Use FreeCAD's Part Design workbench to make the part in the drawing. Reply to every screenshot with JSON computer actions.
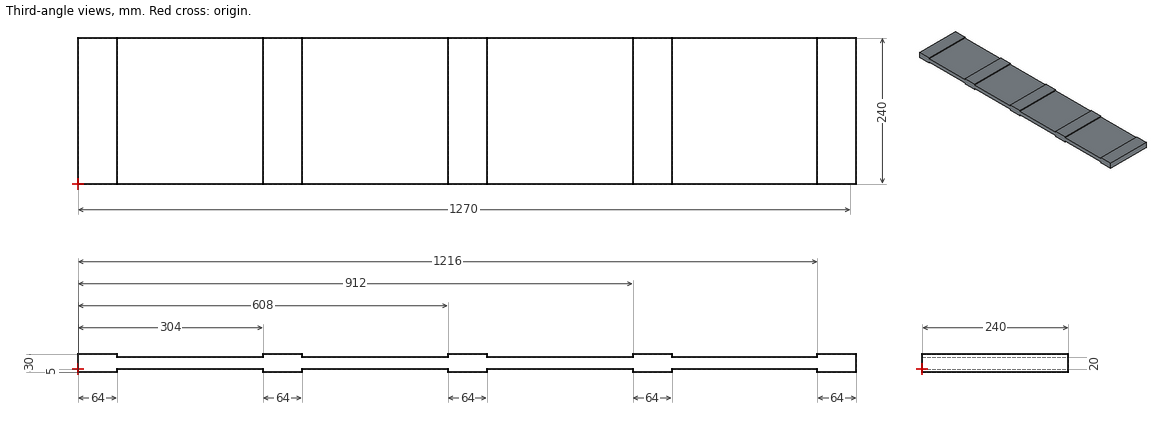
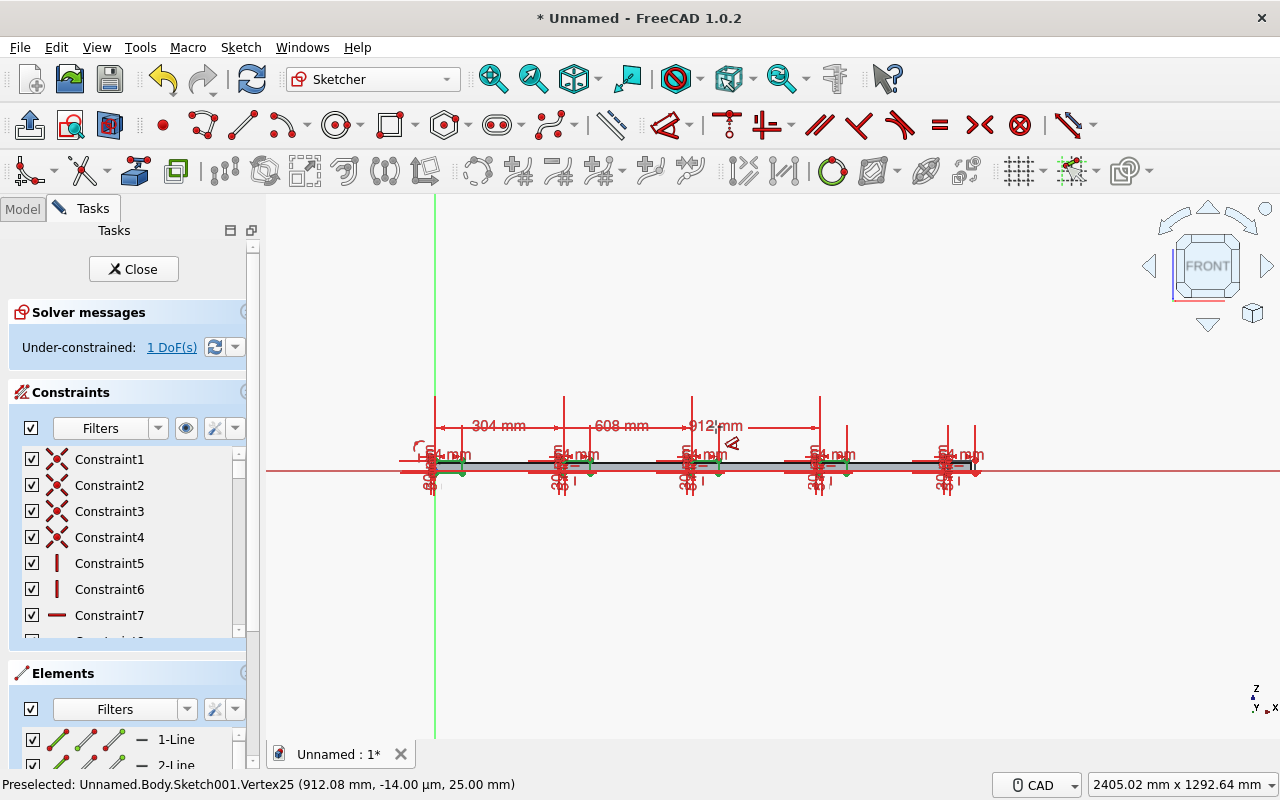
{"action": "left_click", "coordinate": [948, 461]}
{"action": "left_click", "coordinate": [810, 427]}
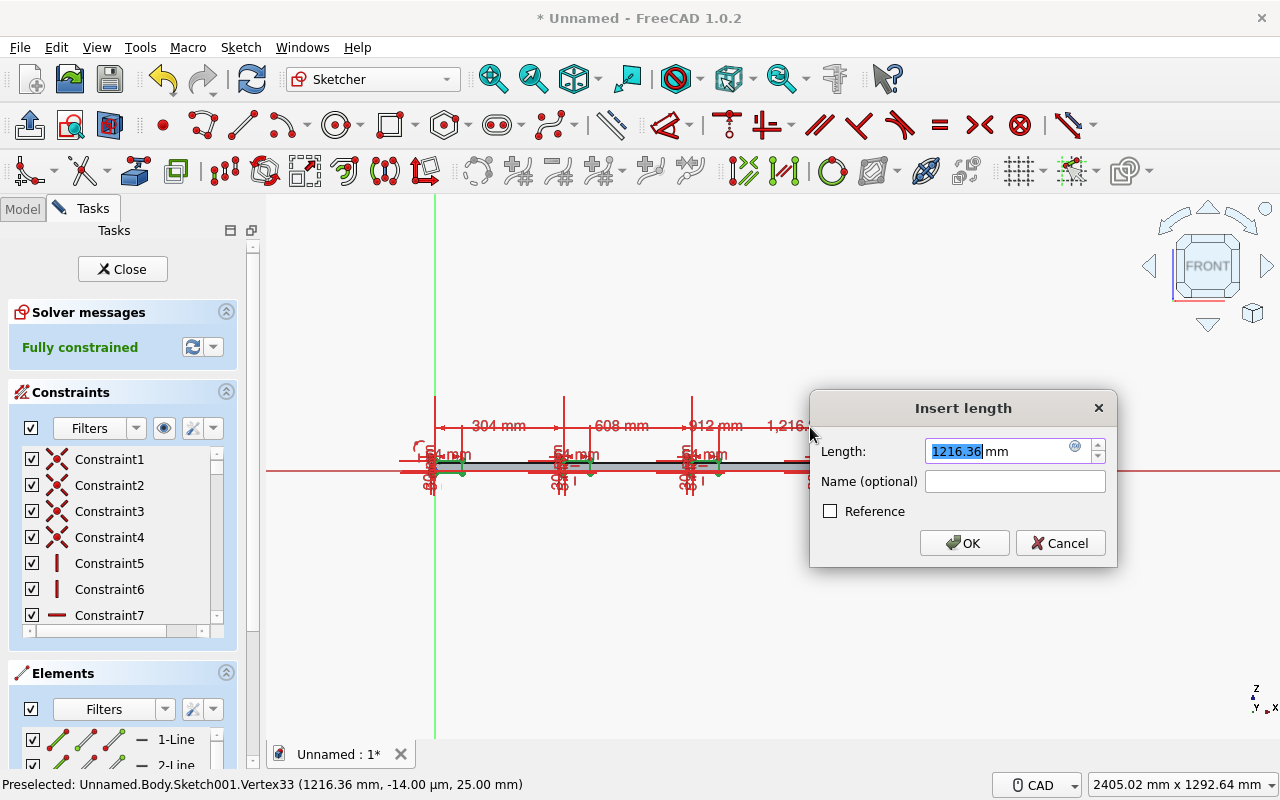
{"action": "type", "text": "1216"}
{"action": "key", "text": "Return"}
{"action": "key", "text": "Escape"}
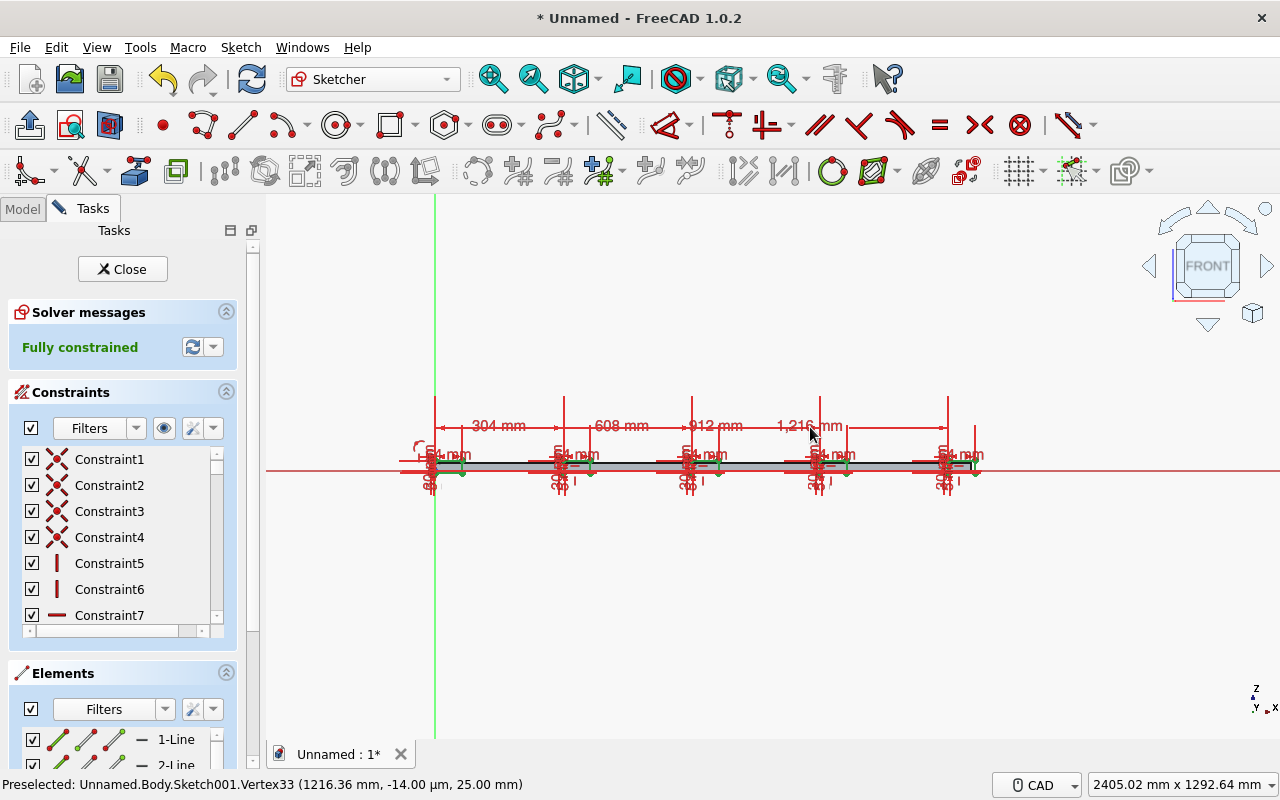
{"action": "left_click", "coordinate": [123, 269]}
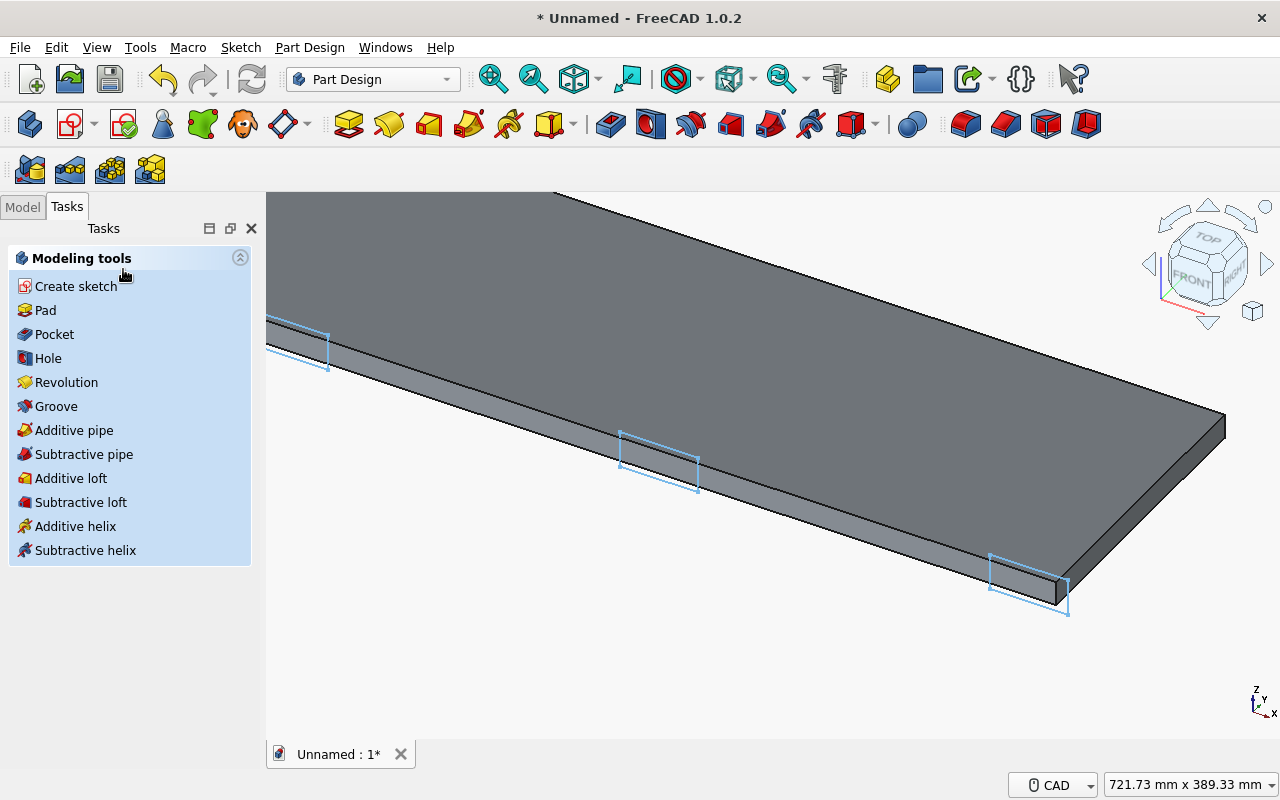
{"action": "left_click", "coordinate": [350, 124]}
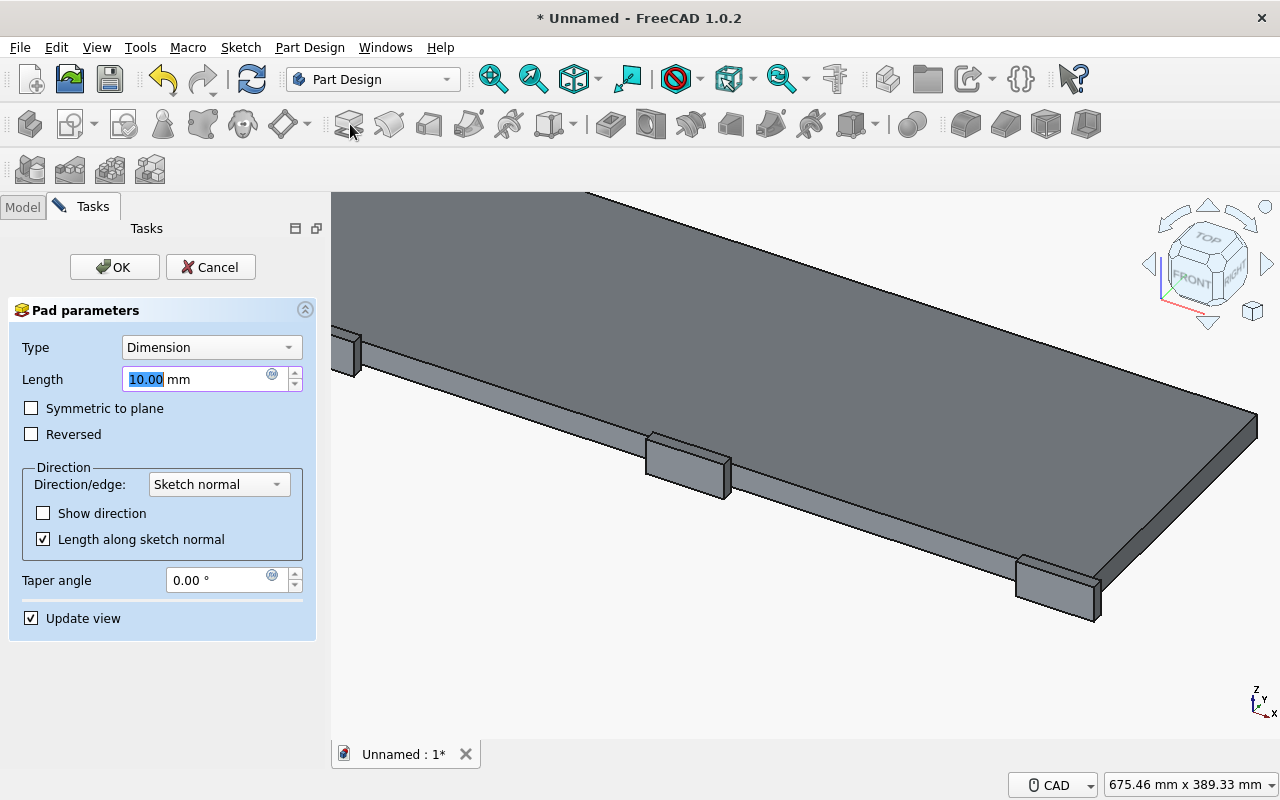
{"action": "type", "text": "240"}
{"action": "key", "text": "Tab"}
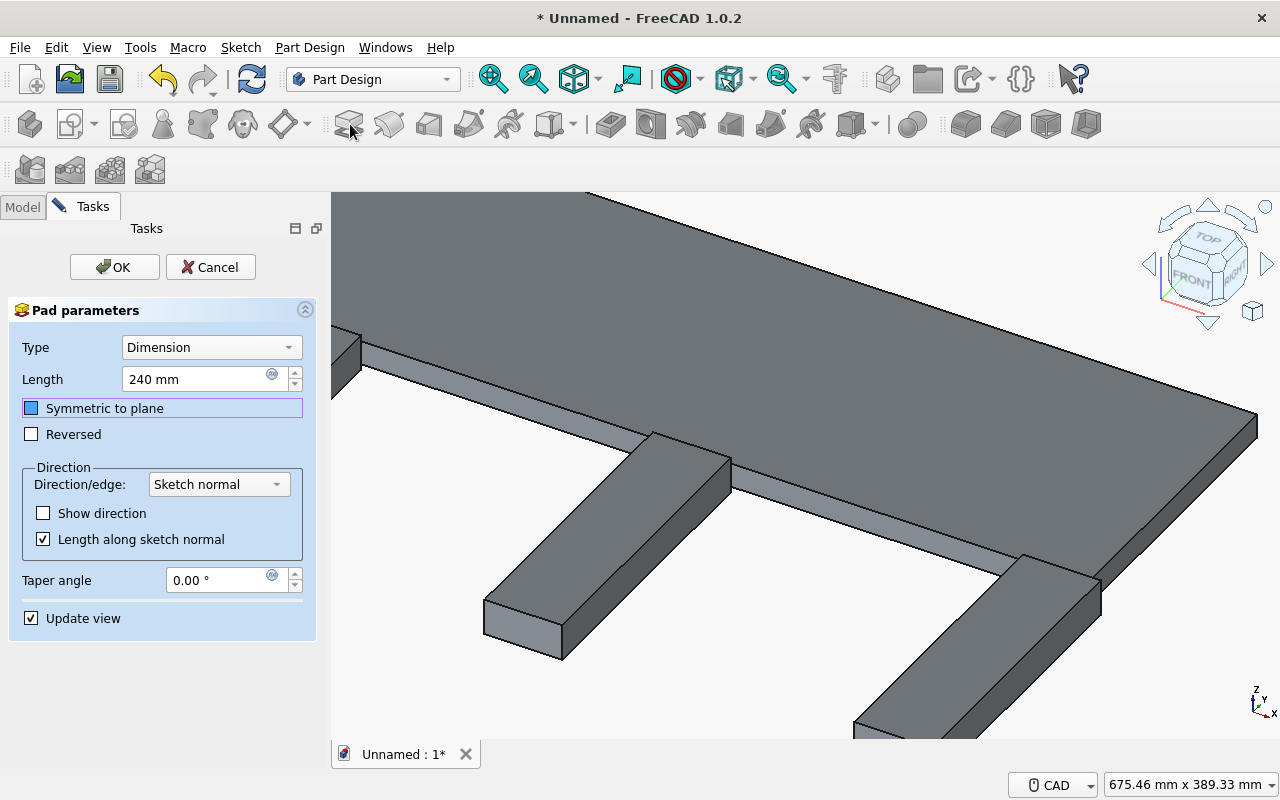
{"action": "left_click", "coordinate": [30, 434]}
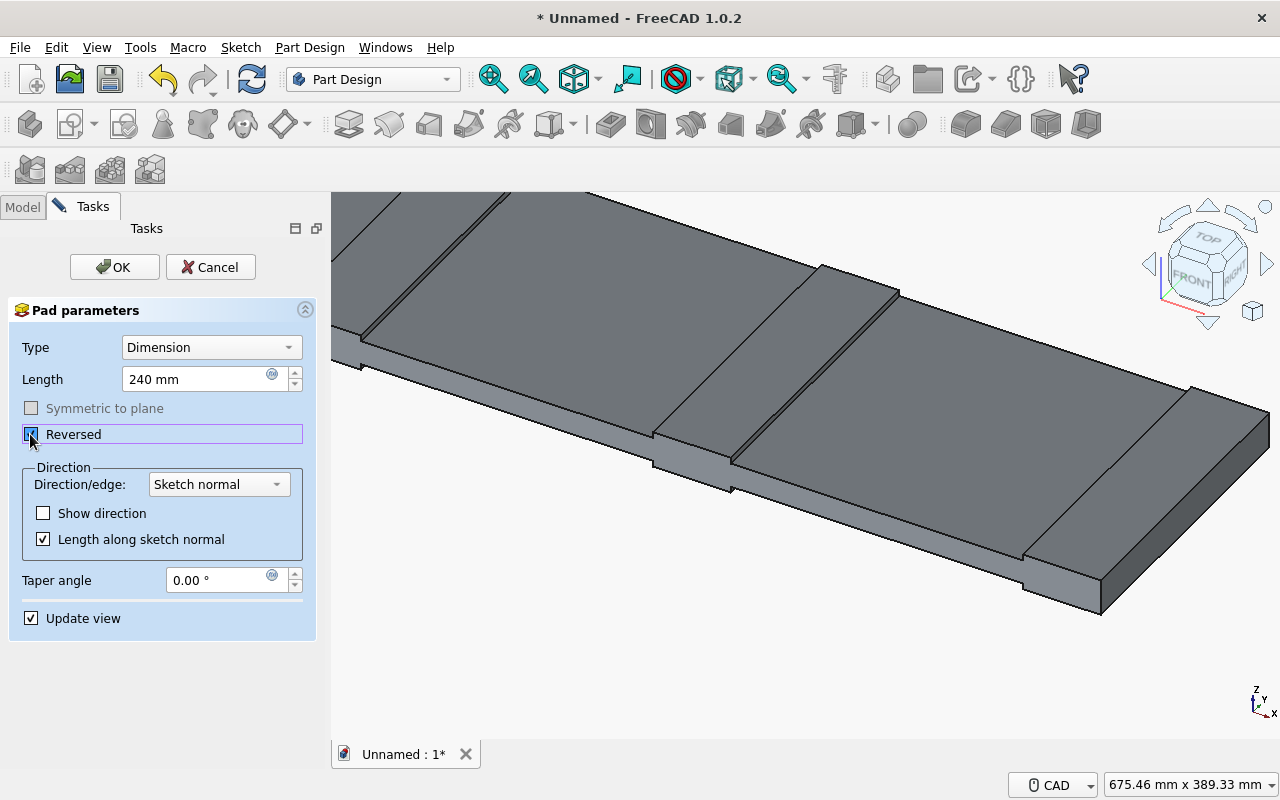
{"action": "left_click", "coordinate": [115, 267]}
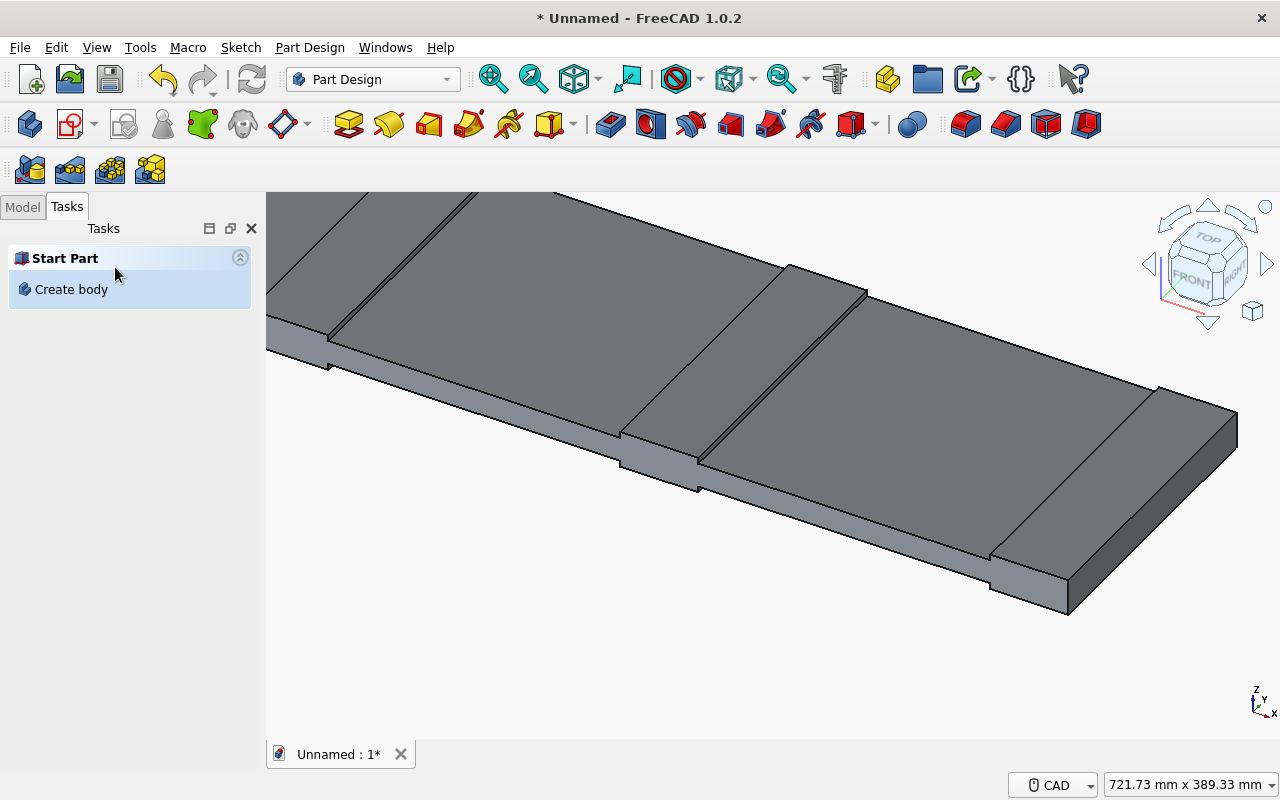
{"action": "key", "text": "0"}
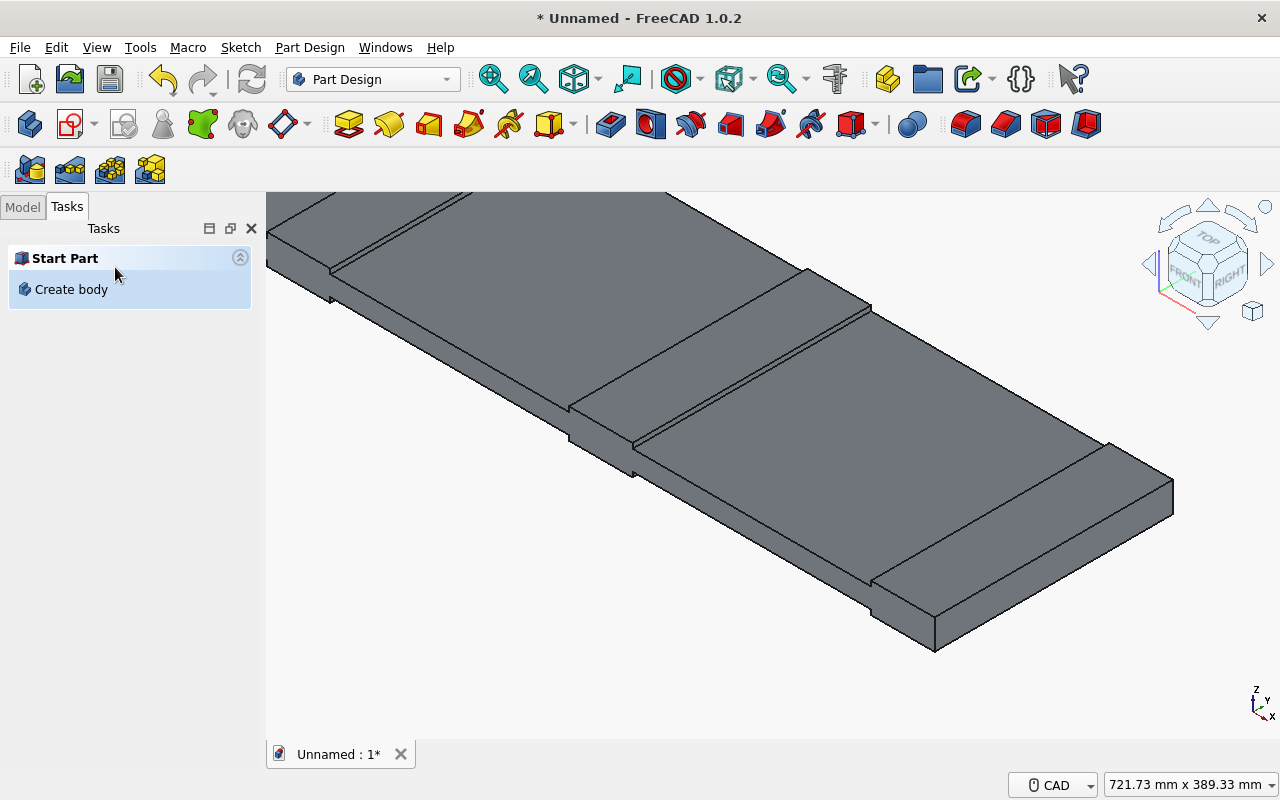
{"action": "key", "text": "v f"}